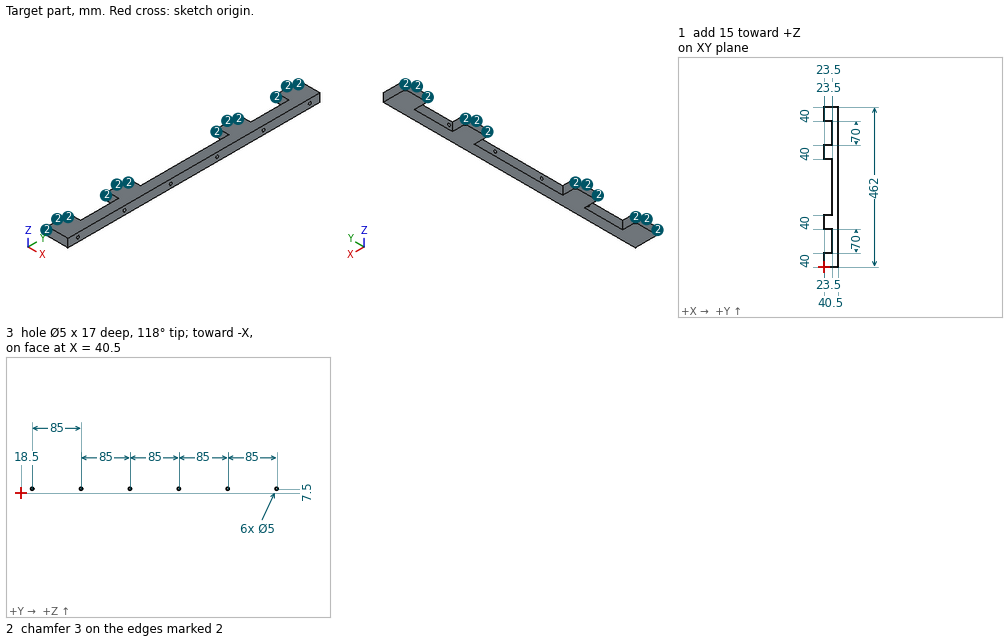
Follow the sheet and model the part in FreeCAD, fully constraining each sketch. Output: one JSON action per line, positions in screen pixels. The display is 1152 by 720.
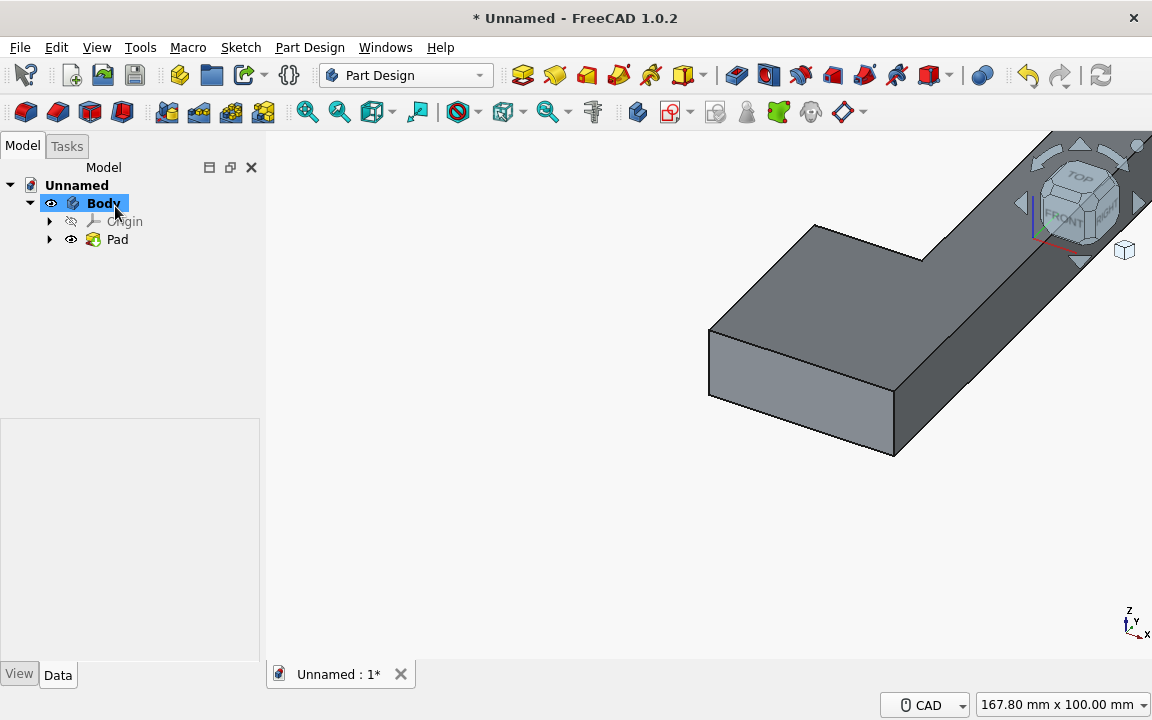
{"action": "key", "text": "v f"}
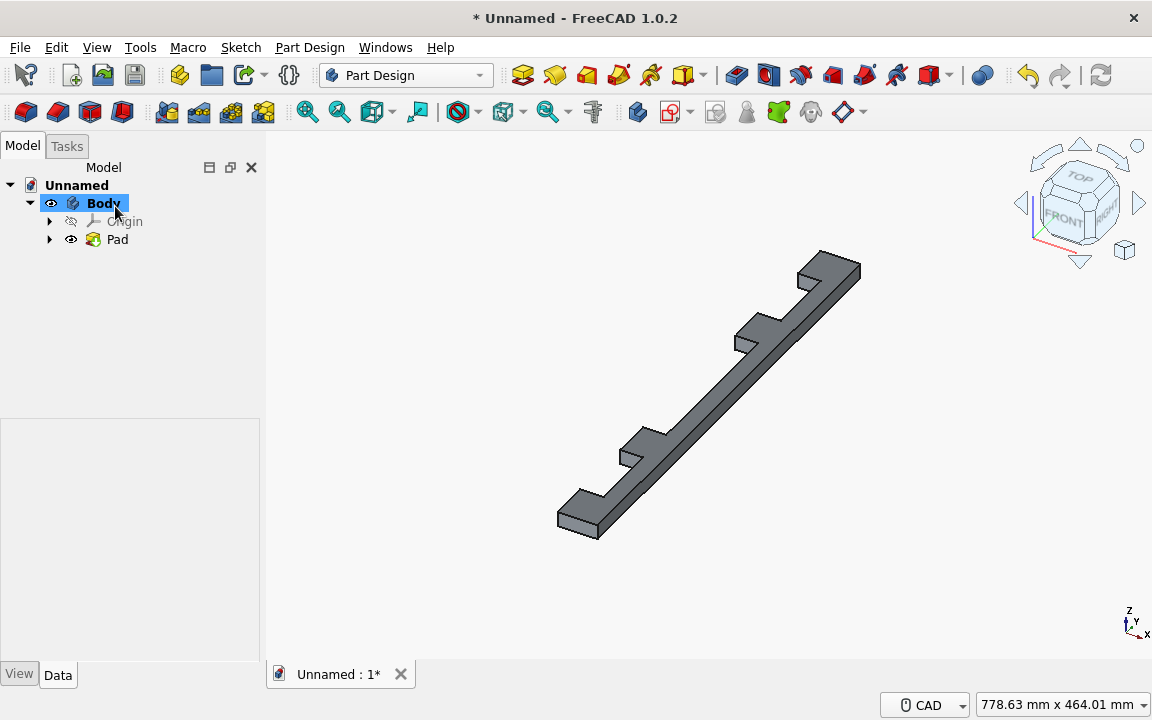
{"action": "key", "text": "0"}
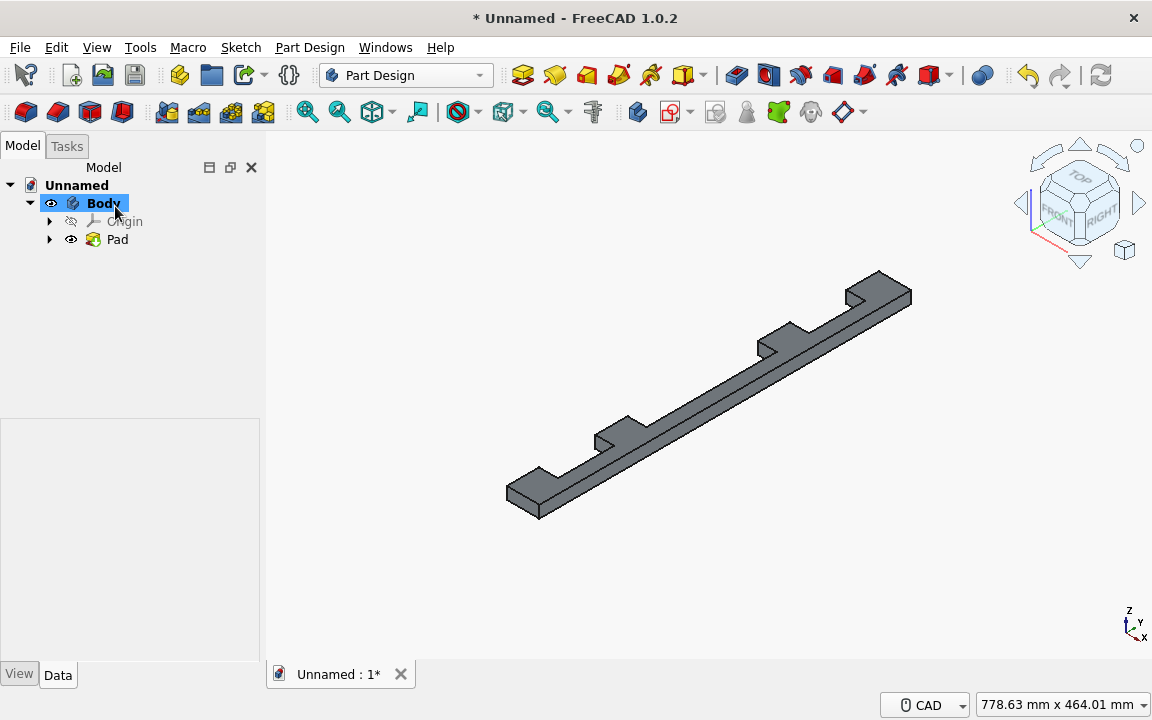
{"action": "key", "text": "2"}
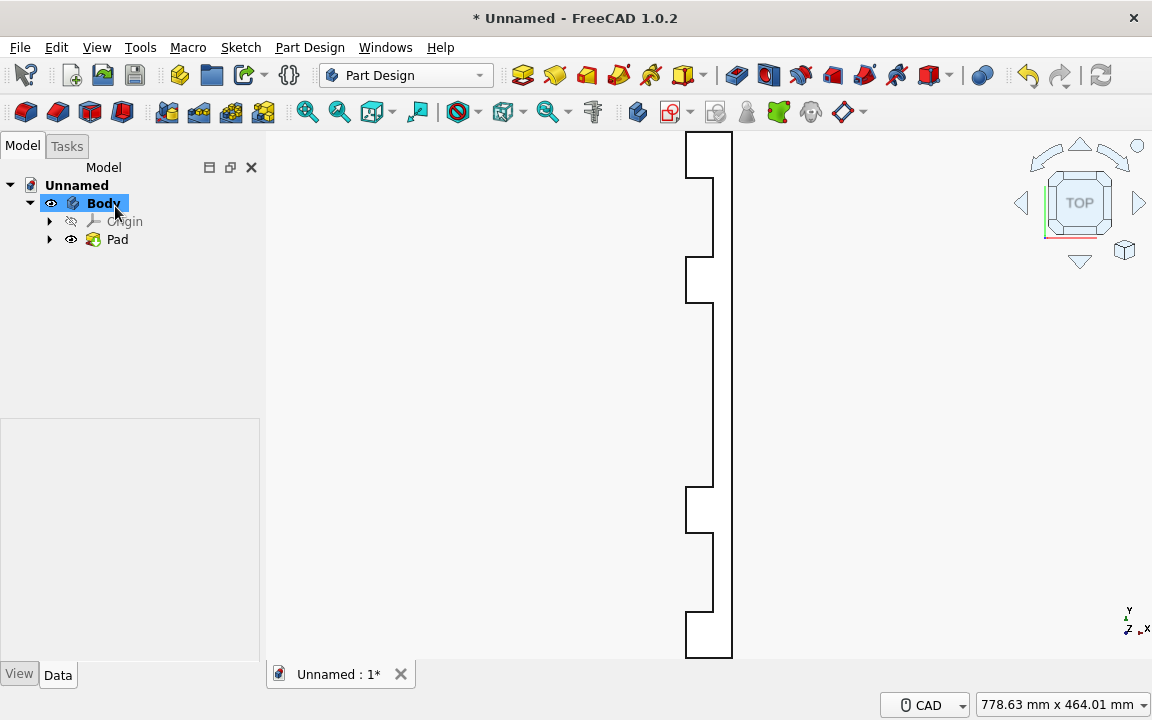
{"action": "left_click", "coordinate": [686, 630]}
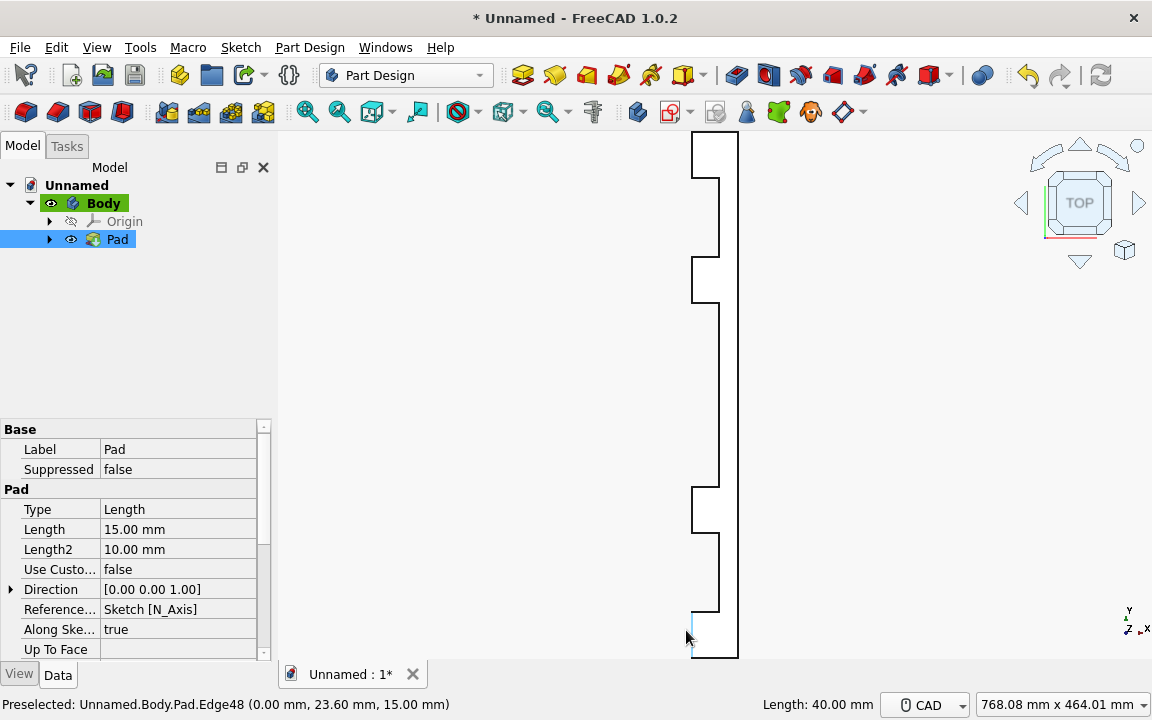
{"action": "left_click", "coordinate": [692, 163], "text": "ctrl"}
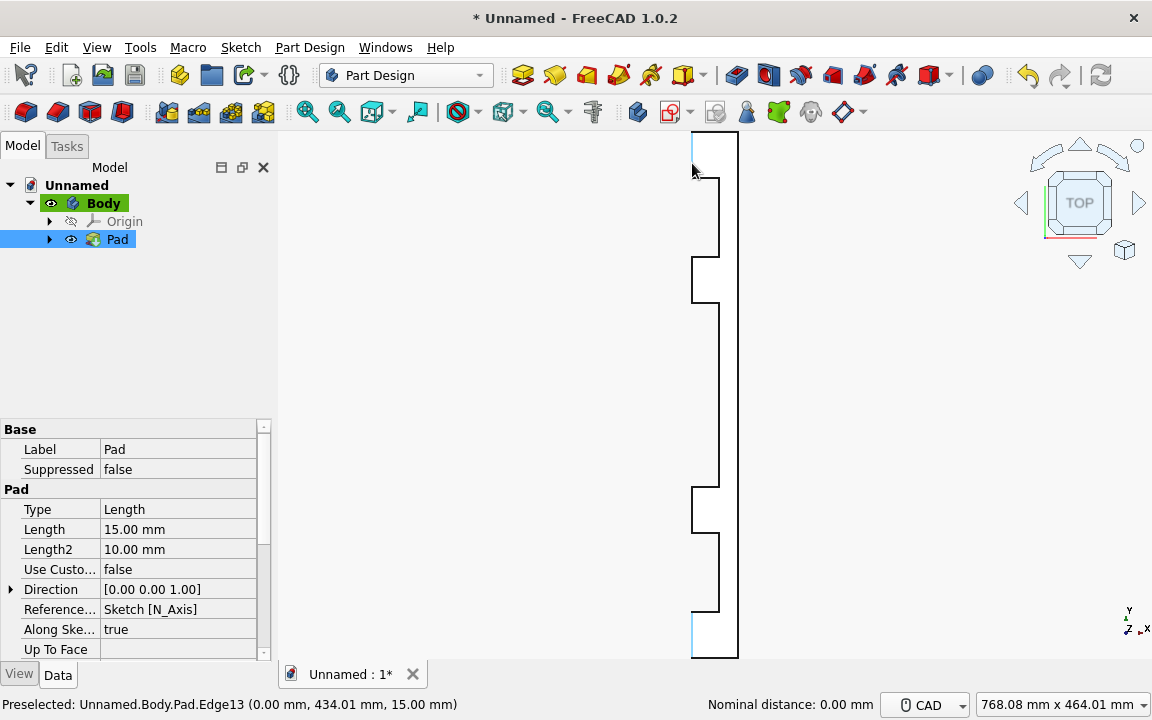
{"action": "left_click", "coordinate": [692, 279], "text": "ctrl"}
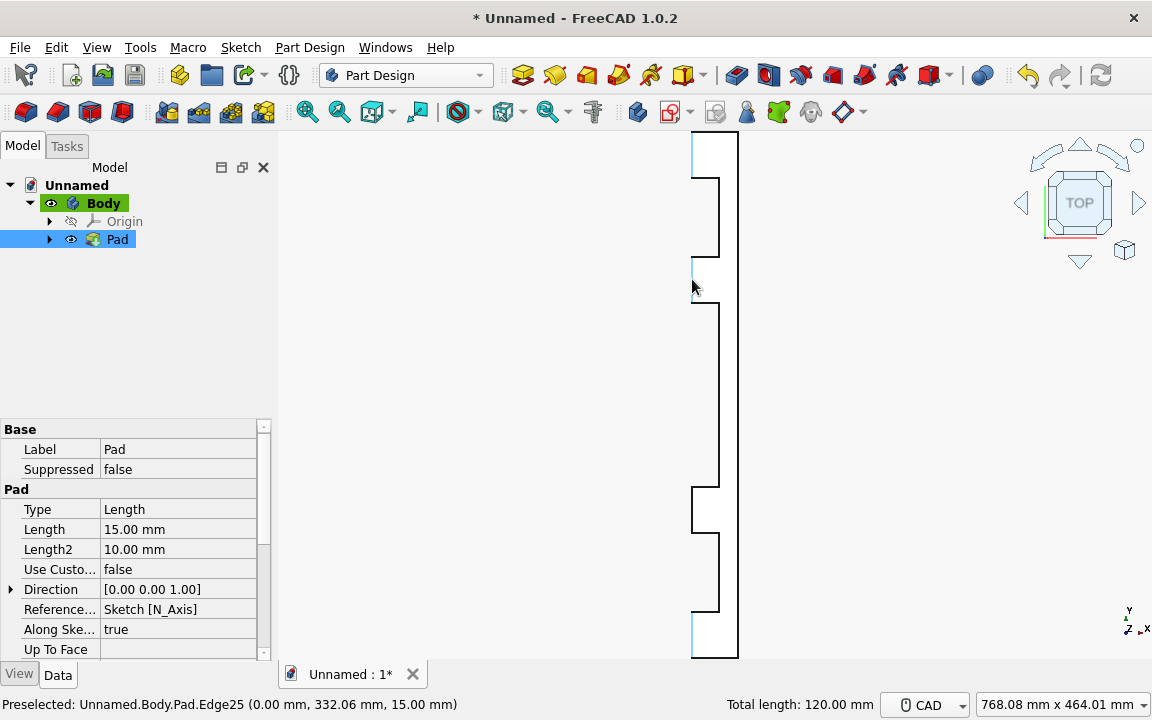
{"action": "left_click", "coordinate": [692, 509], "text": "ctrl"}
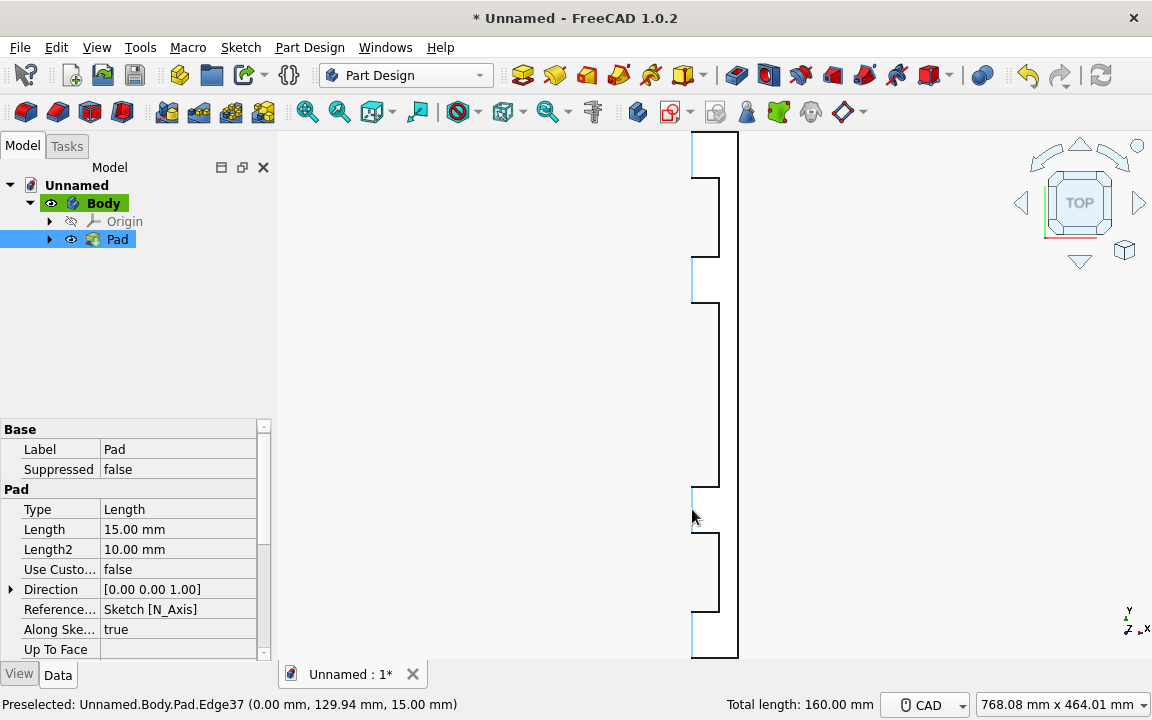
{"action": "scroll", "coordinate": [692, 532], "scroll_direction": "up", "scroll_amount": 5}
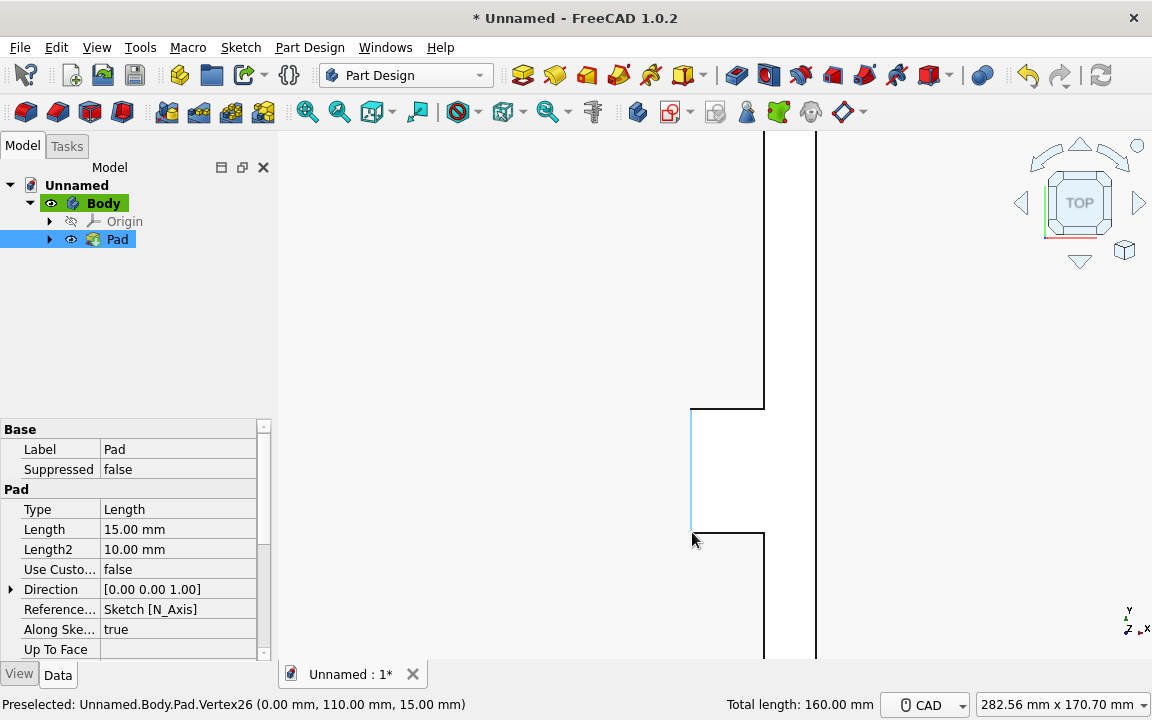
{"action": "left_click", "coordinate": [308, 112]}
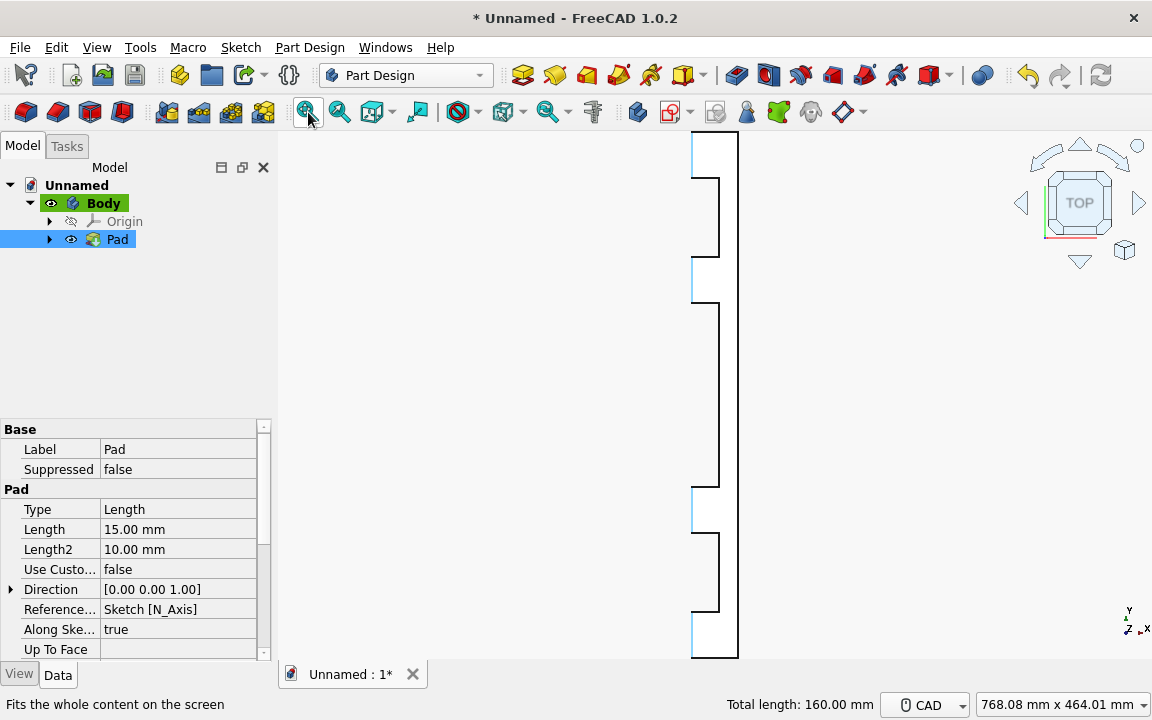
{"action": "key", "text": "1"}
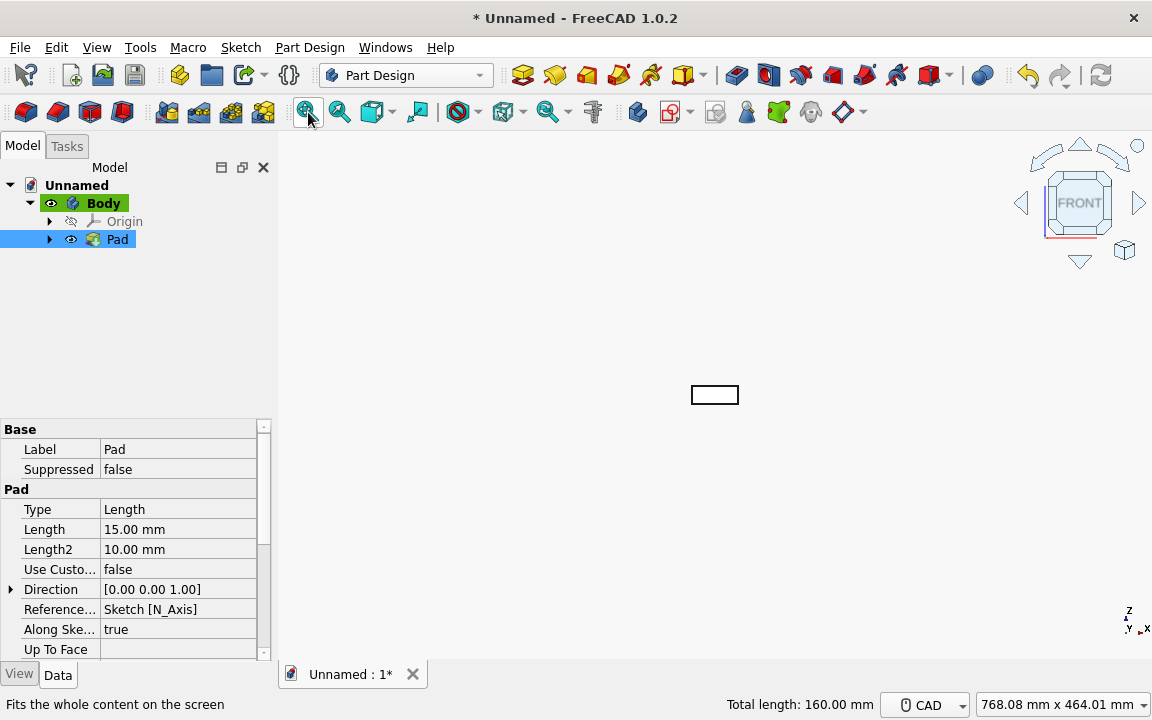
{"action": "left_click", "coordinate": [308, 112]}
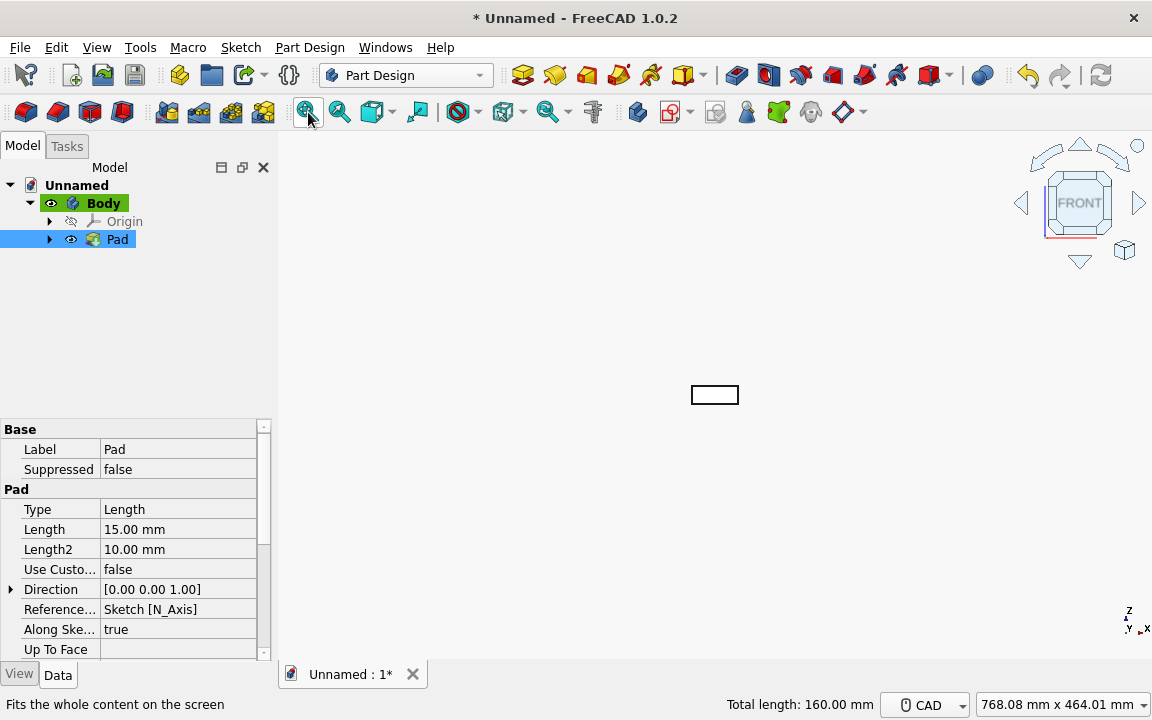
{"action": "left_click", "coordinate": [692, 394], "text": "ctrl"}